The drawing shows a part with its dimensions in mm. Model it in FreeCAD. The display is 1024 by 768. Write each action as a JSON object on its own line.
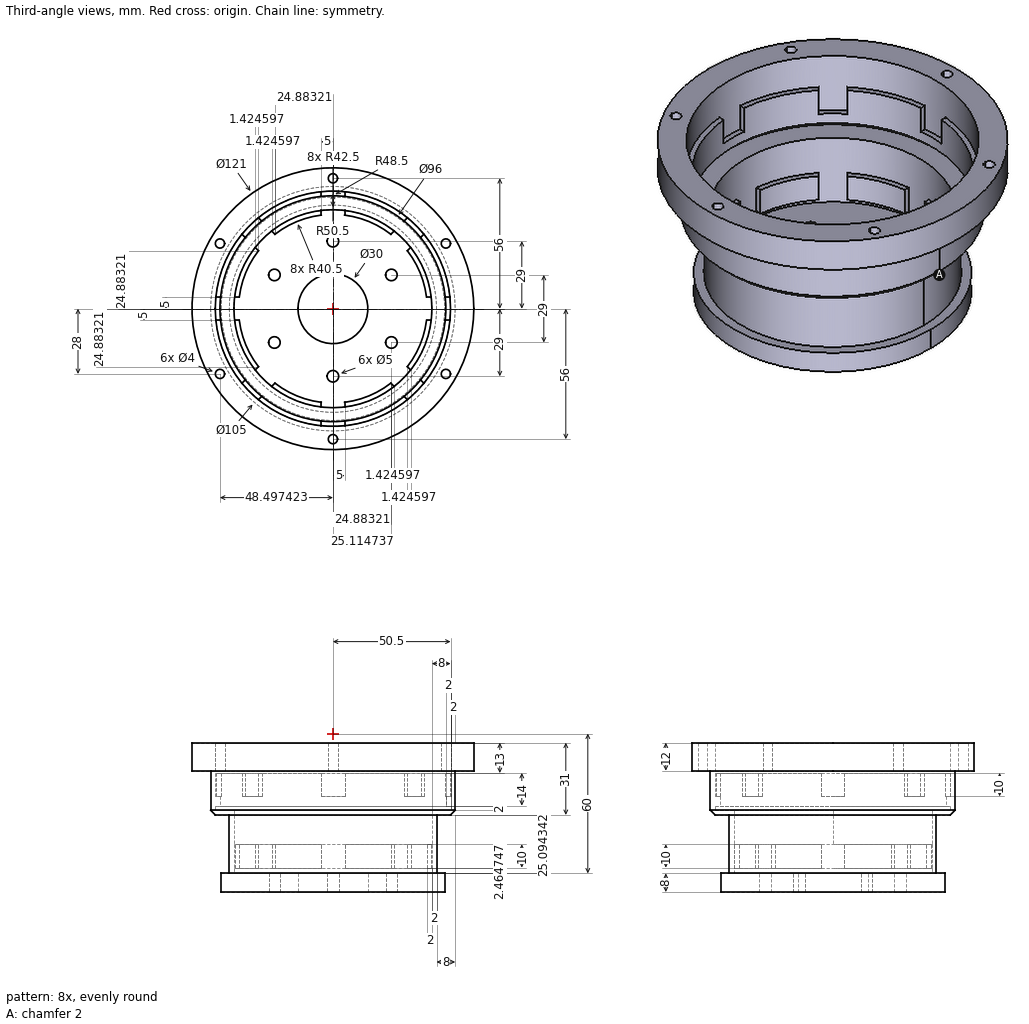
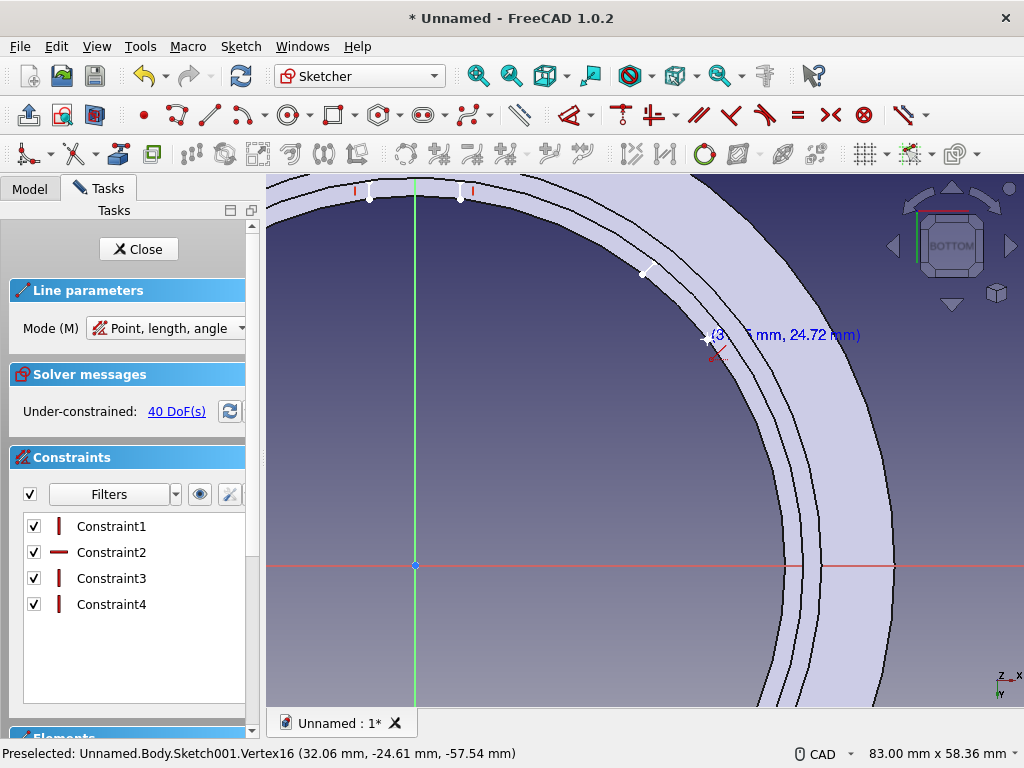
{"action": "left_click", "coordinate": [782, 520]}
{"action": "left_click", "coordinate": [801, 520]}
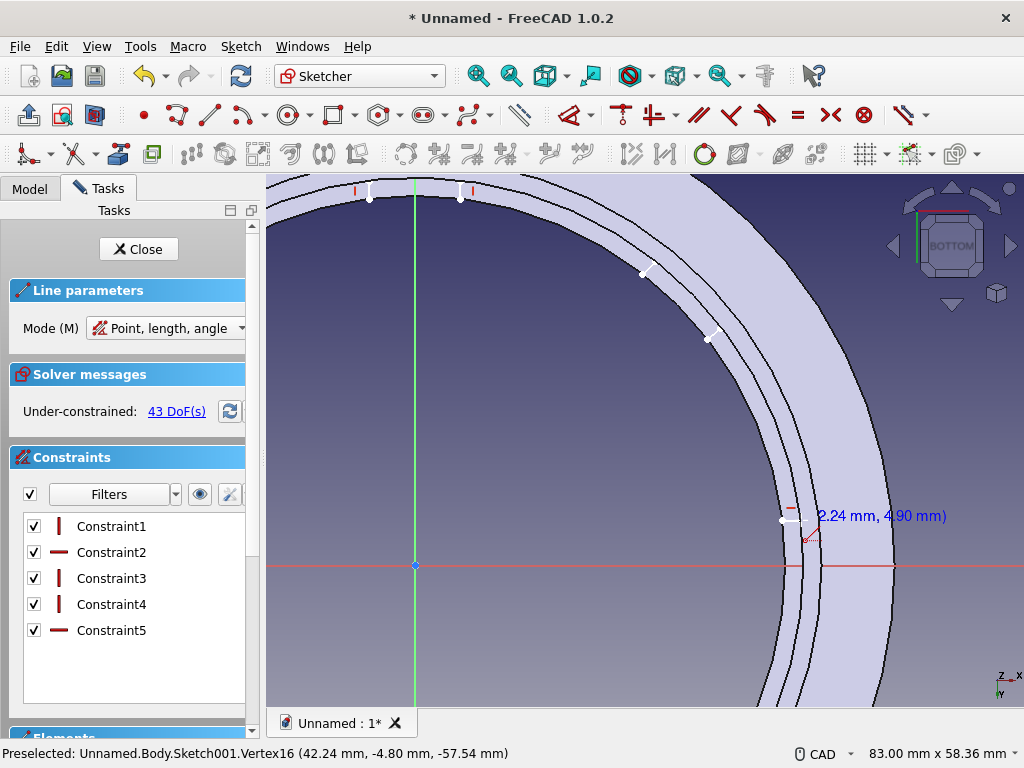
{"action": "left_click", "coordinate": [801, 611]}
{"action": "left_click", "coordinate": [782, 611]}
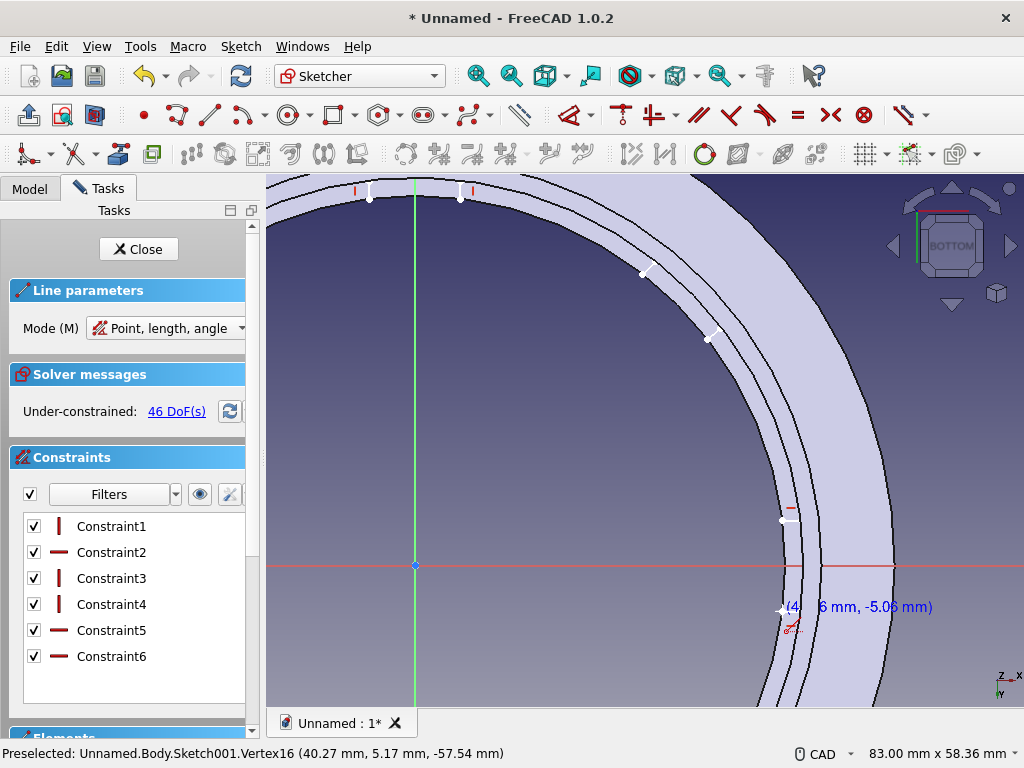
{"action": "scroll", "coordinate": [708, 338], "scroll_direction": "down", "scroll_amount": 4}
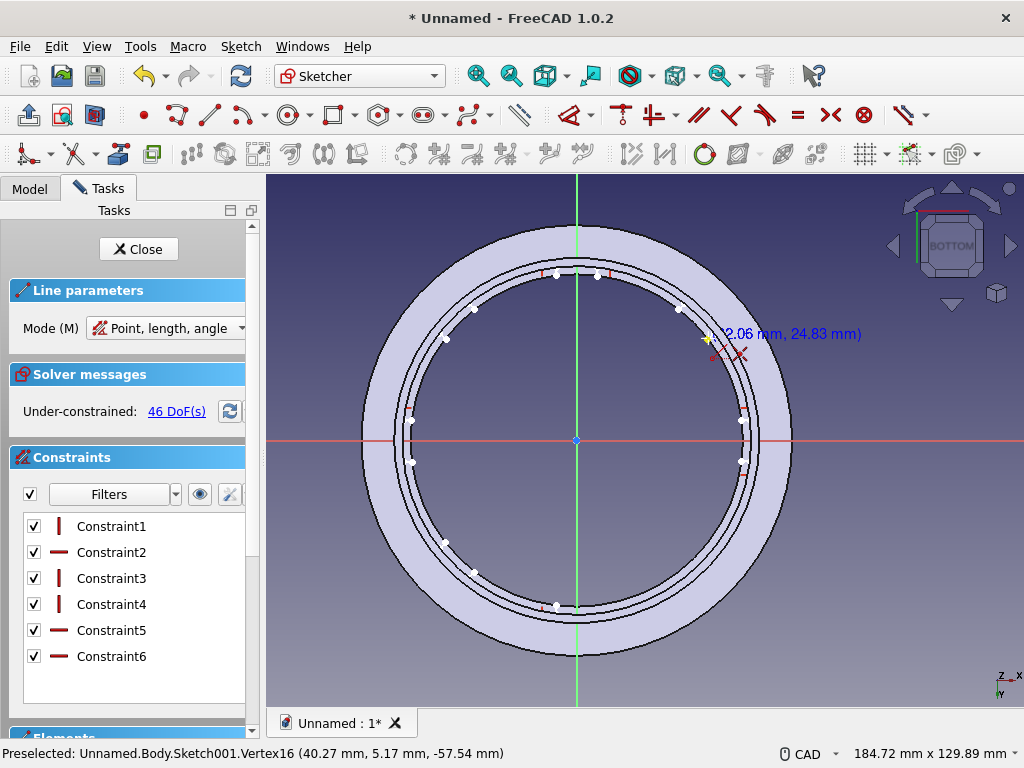
{"action": "left_click", "coordinate": [708, 543]}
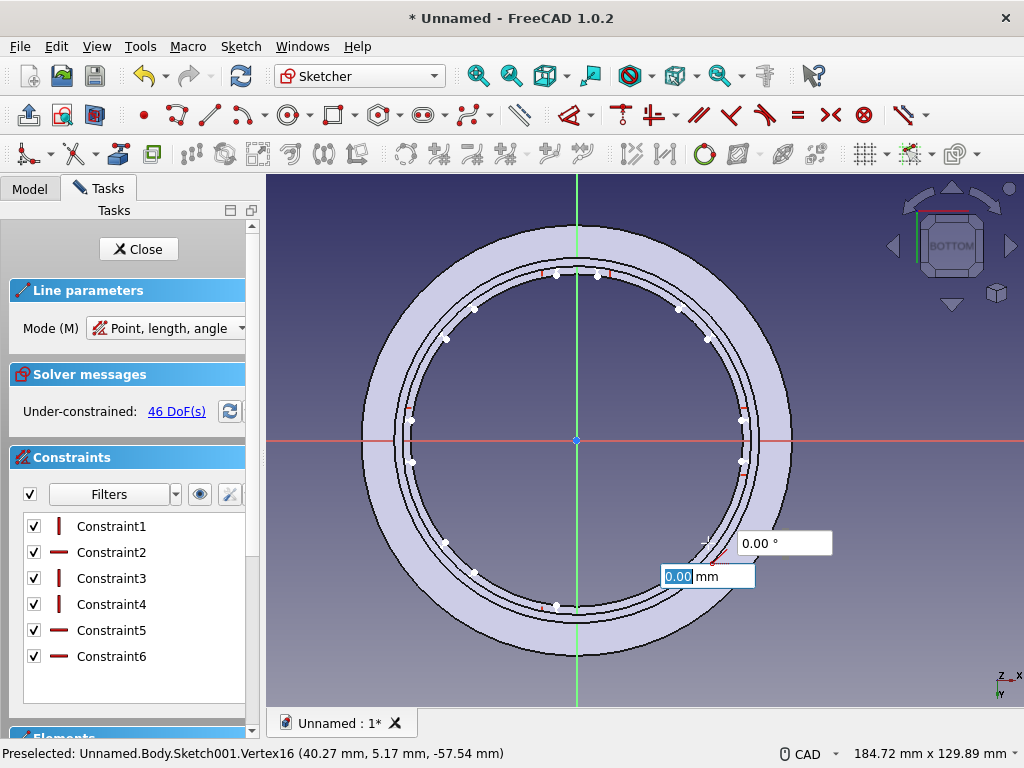
{"action": "scroll", "coordinate": [714, 548], "scroll_direction": "up", "scroll_amount": 4}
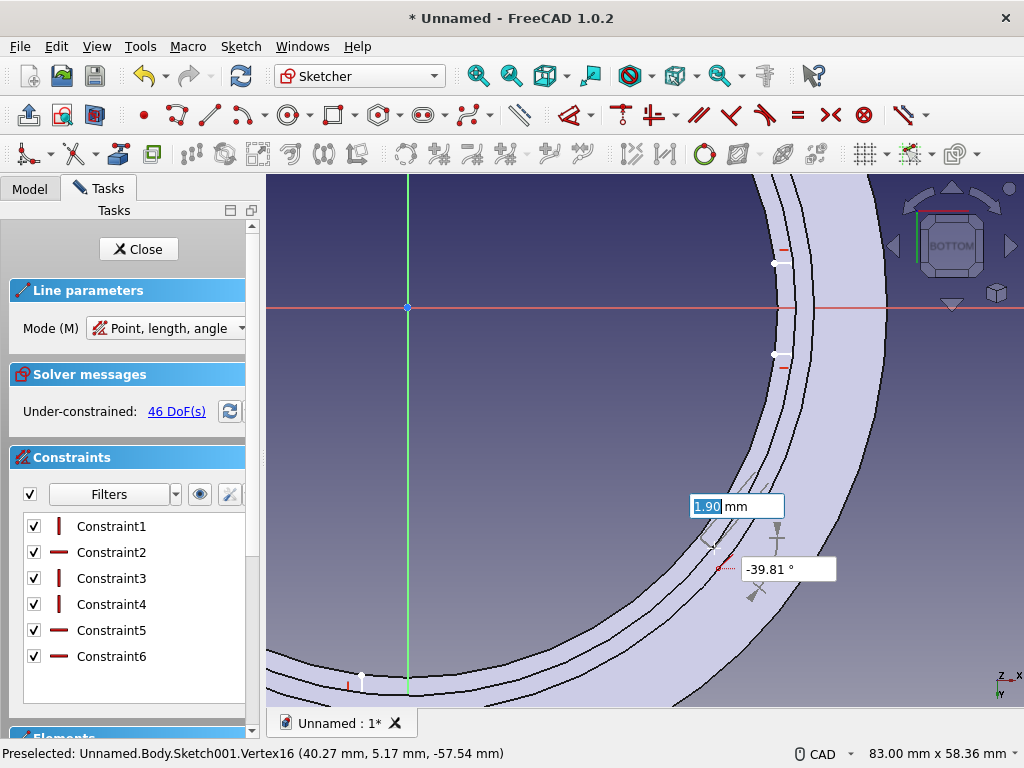
{"action": "left_click", "coordinate": [713, 548]}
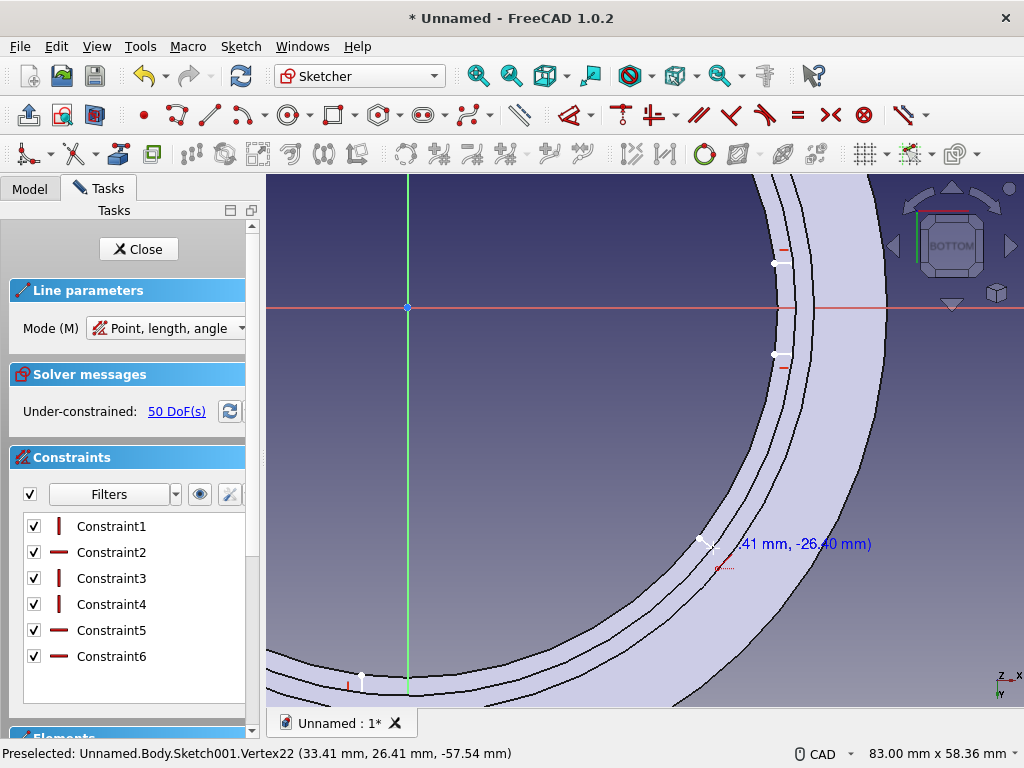
{"action": "left_click", "coordinate": [648, 613]}
{"action": "left_click", "coordinate": [635, 600]}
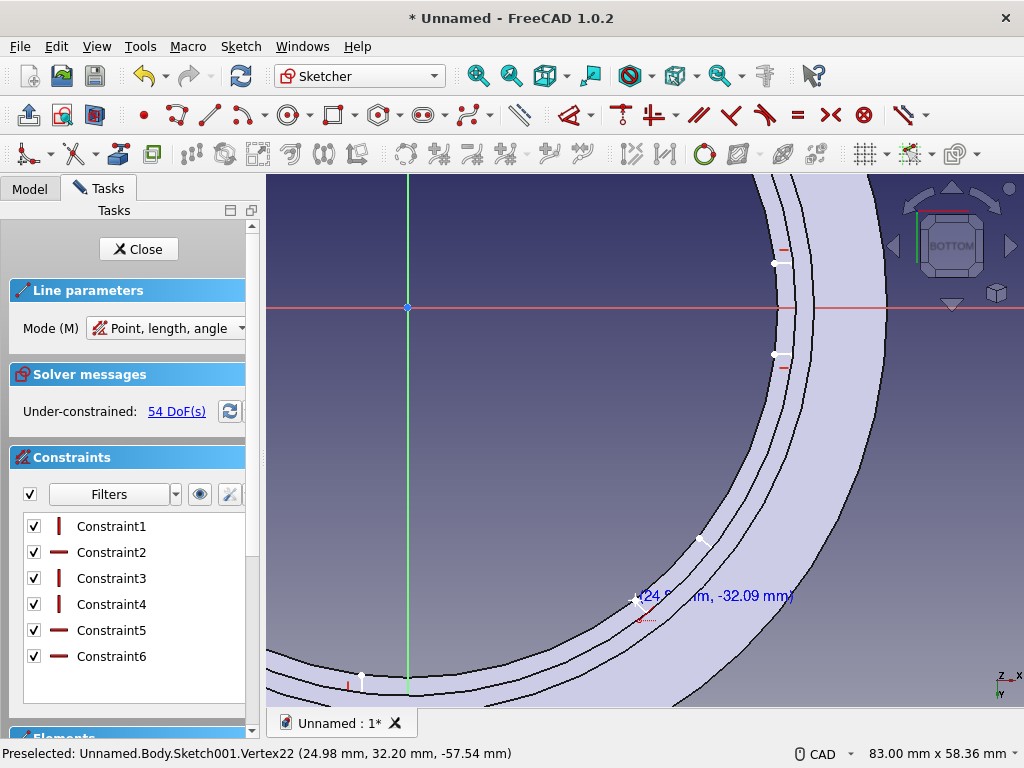
{"action": "left_click", "coordinate": [454, 675]}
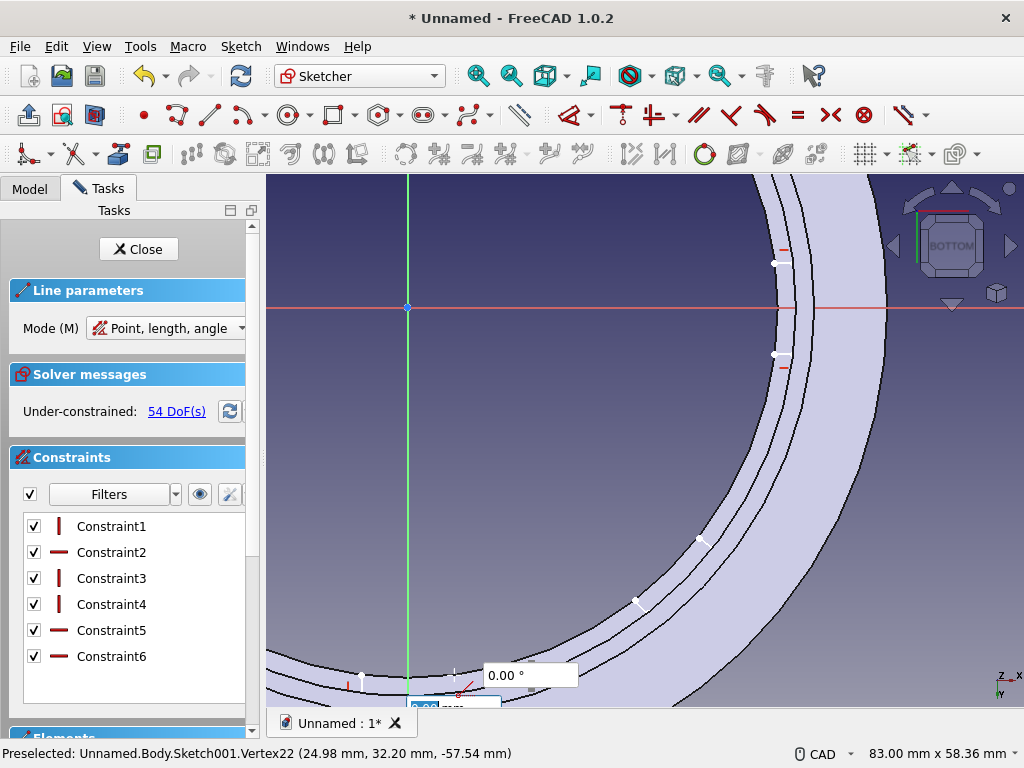
{"action": "scroll", "coordinate": [714, 549], "scroll_direction": "down", "scroll_amount": 4}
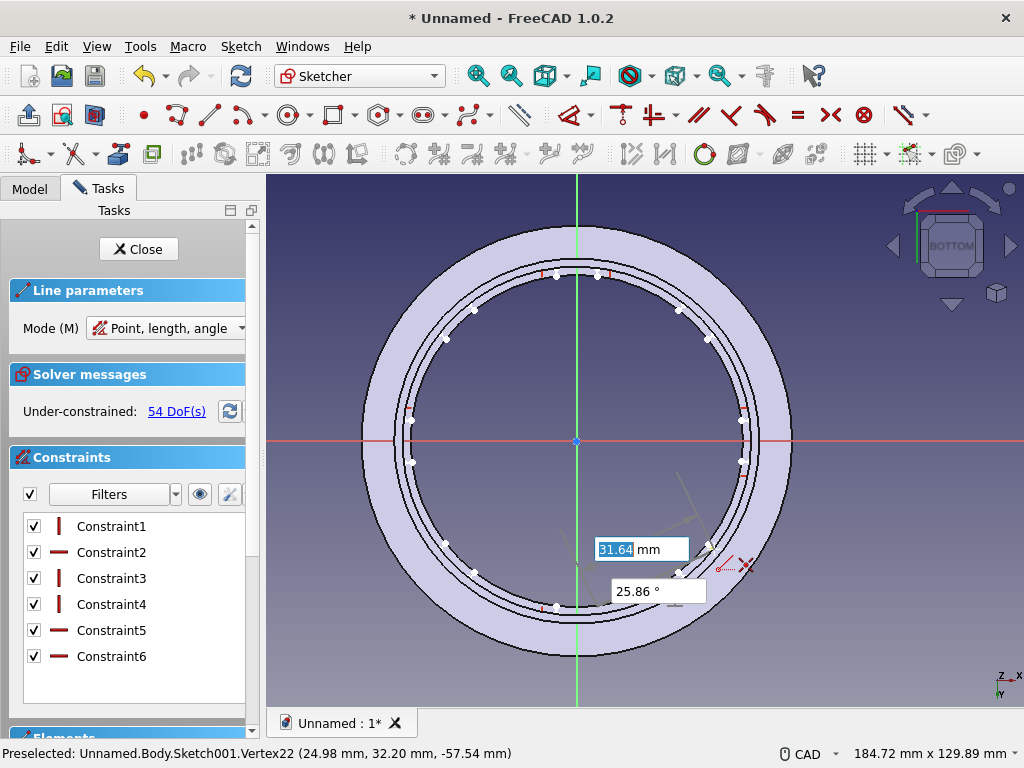
{"action": "scroll", "coordinate": [597, 614], "scroll_direction": "up", "scroll_amount": 4}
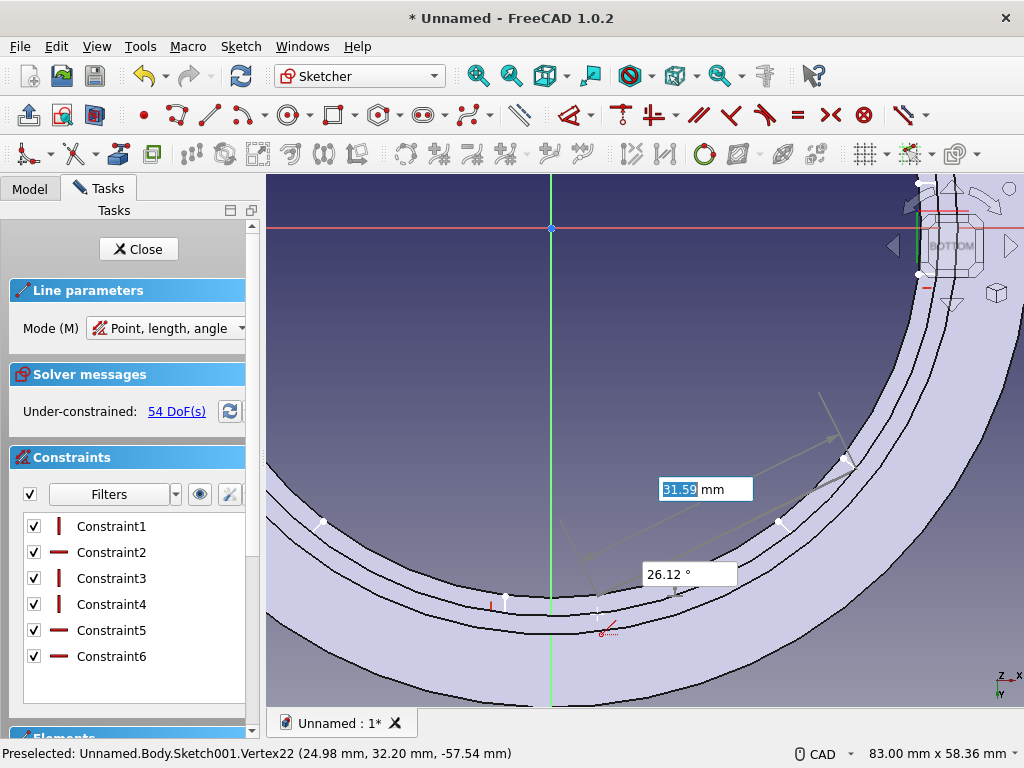
{"action": "left_click", "coordinate": [598, 614]}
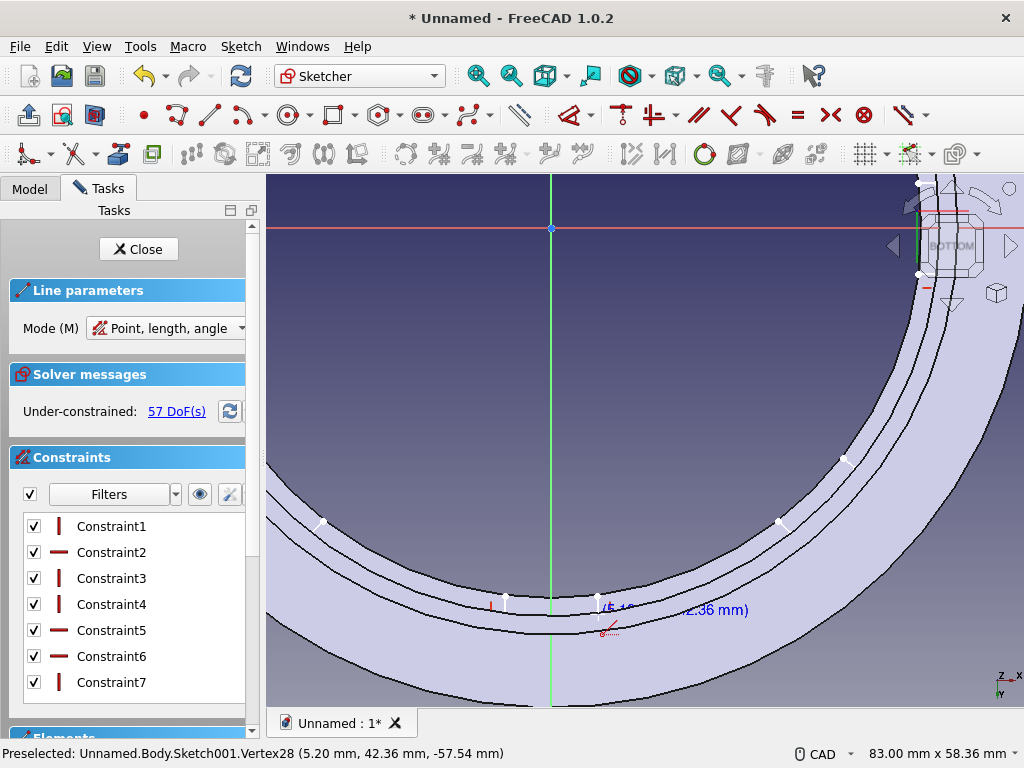
{"action": "key", "text": "g 3 a"}